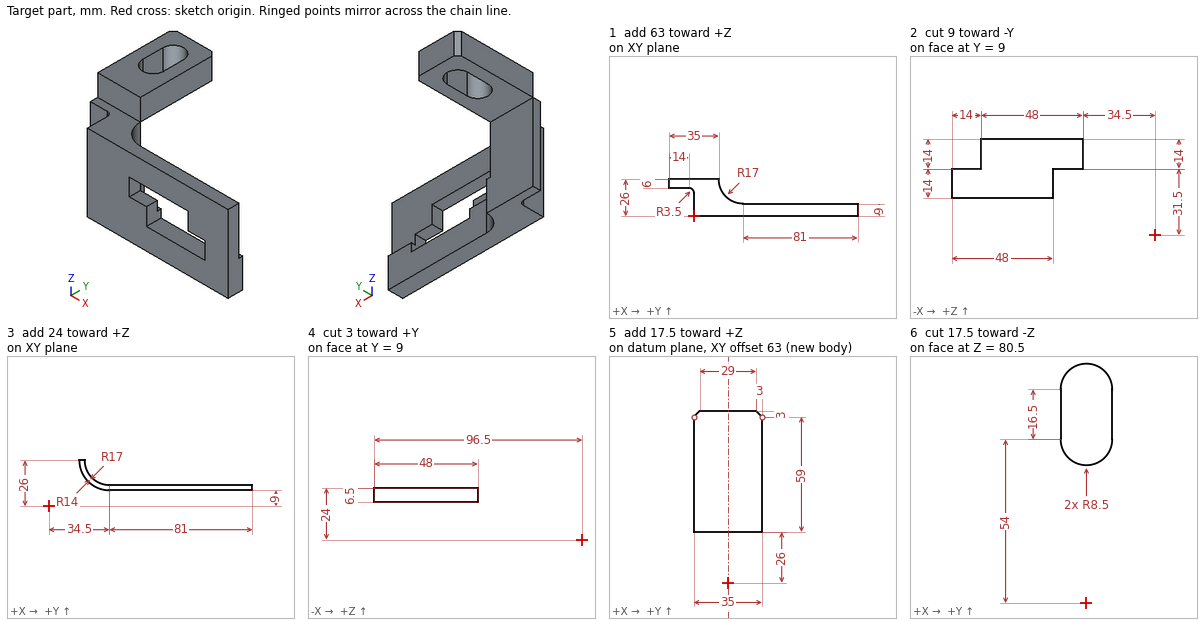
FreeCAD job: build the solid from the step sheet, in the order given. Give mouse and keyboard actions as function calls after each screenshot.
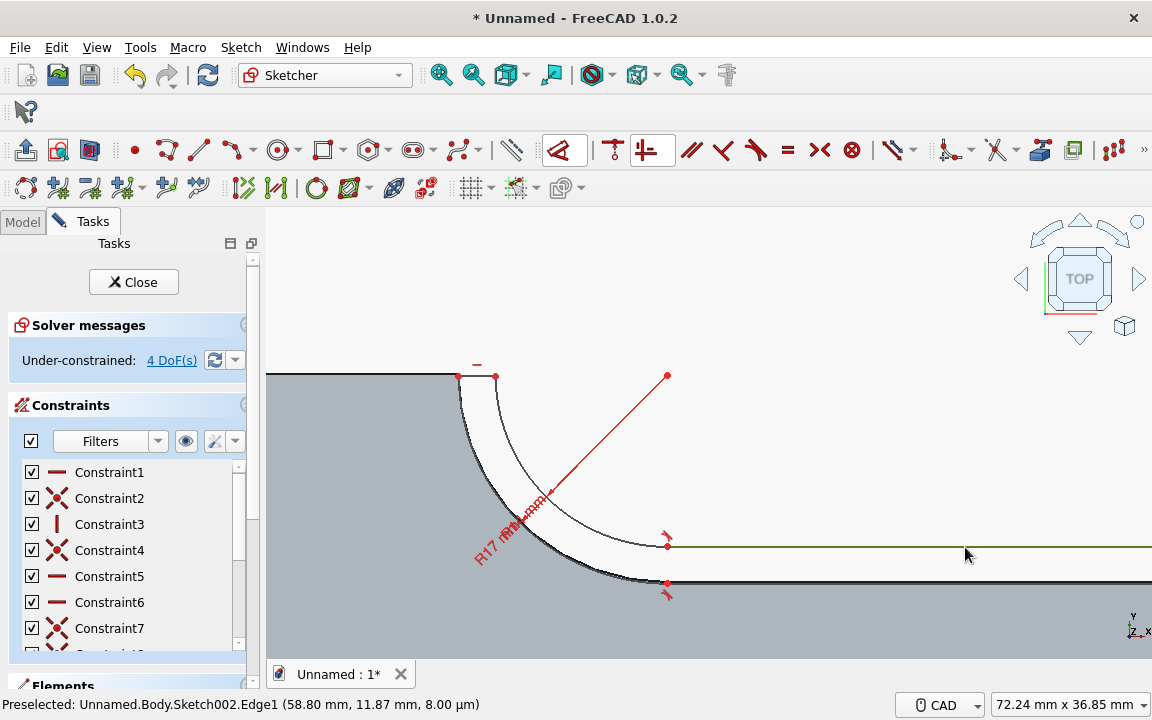
key(l)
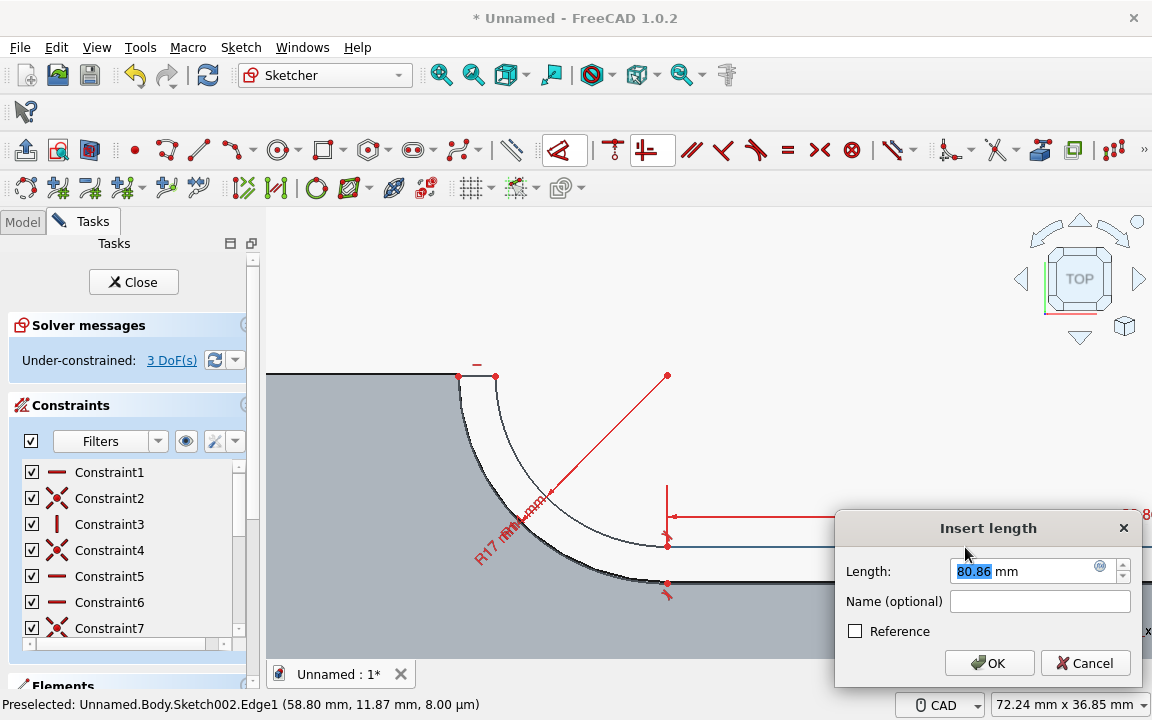
text(81)
key(Return)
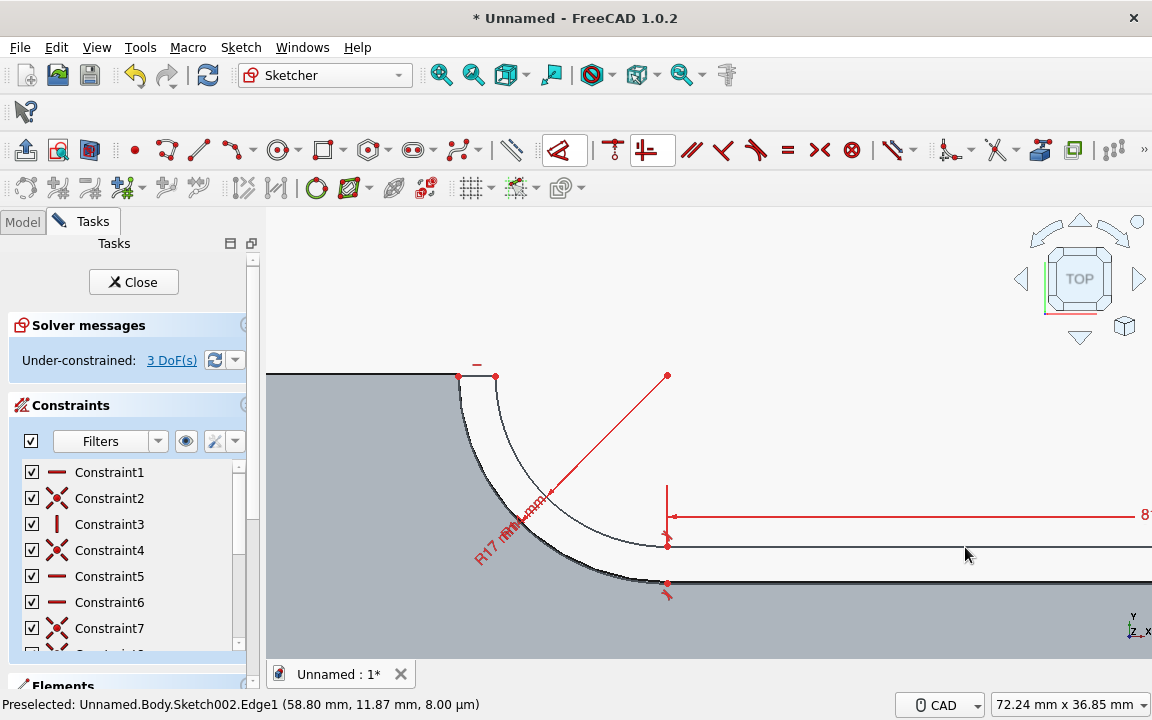
scroll(459, 375, down, 5)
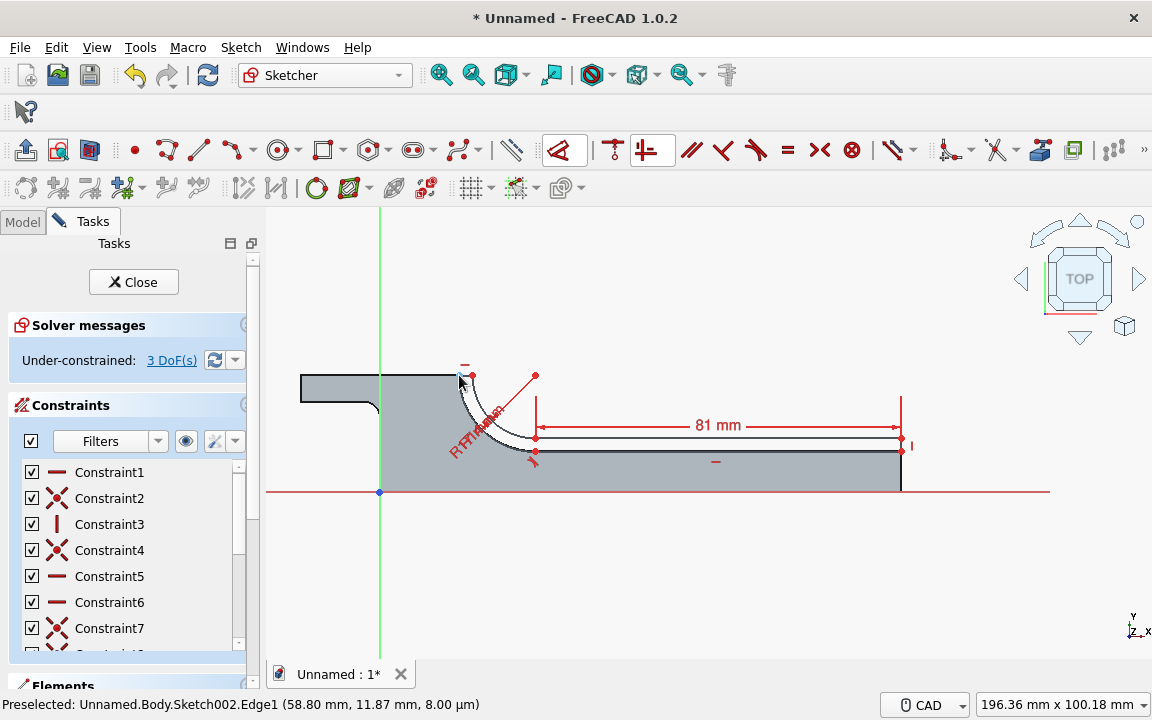
click(901, 452)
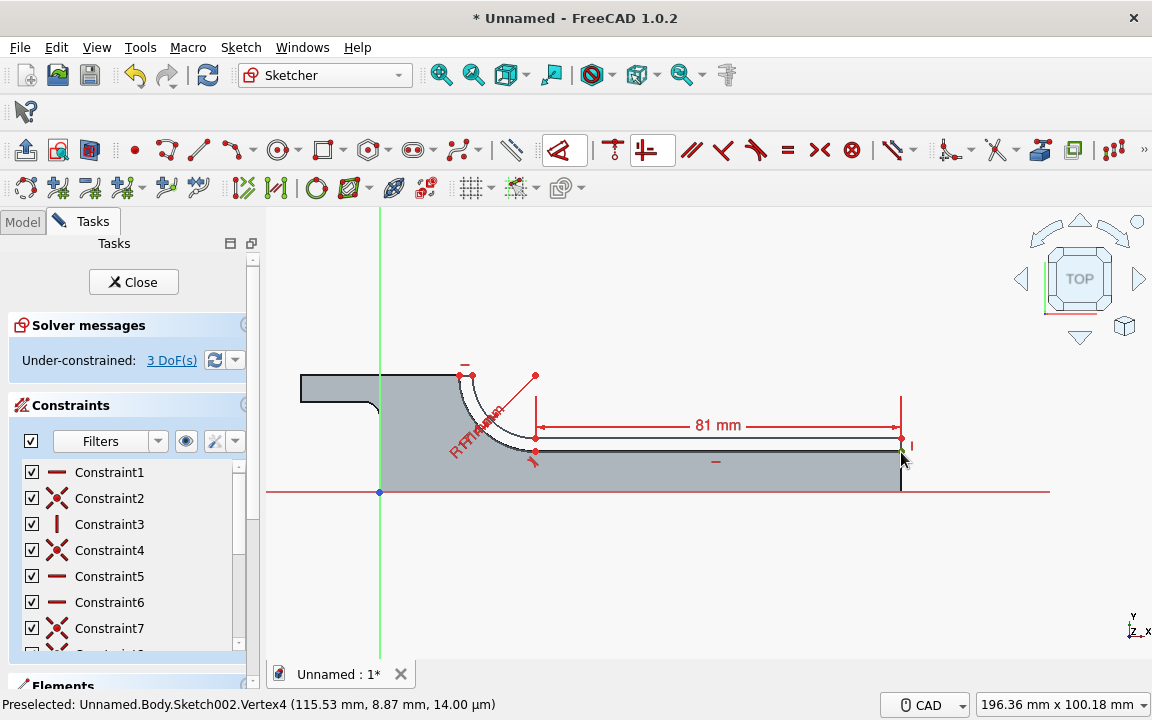
key(i)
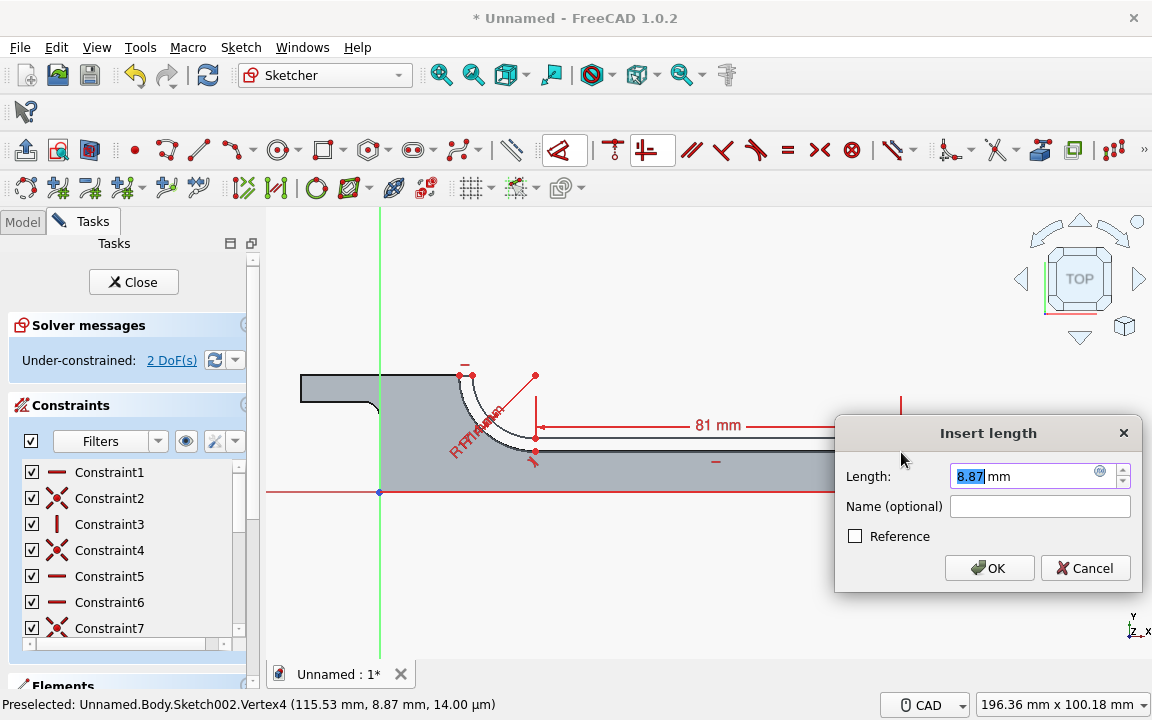
text(9)
key(Return)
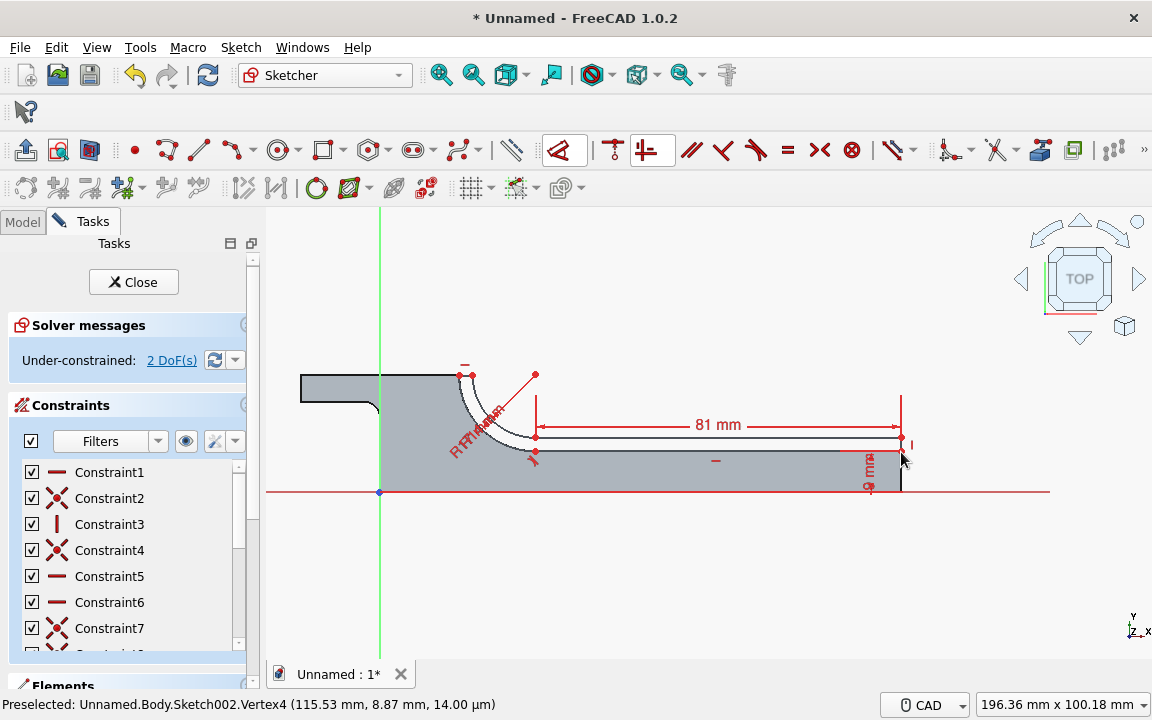
click(459, 376)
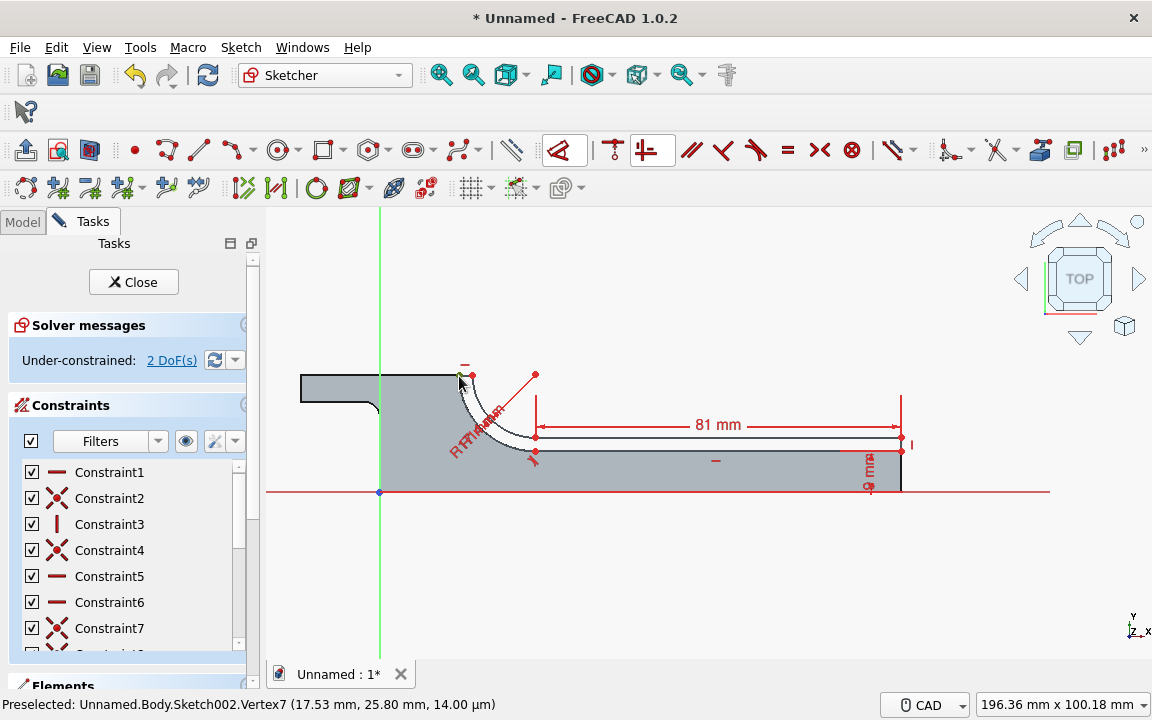
key(i)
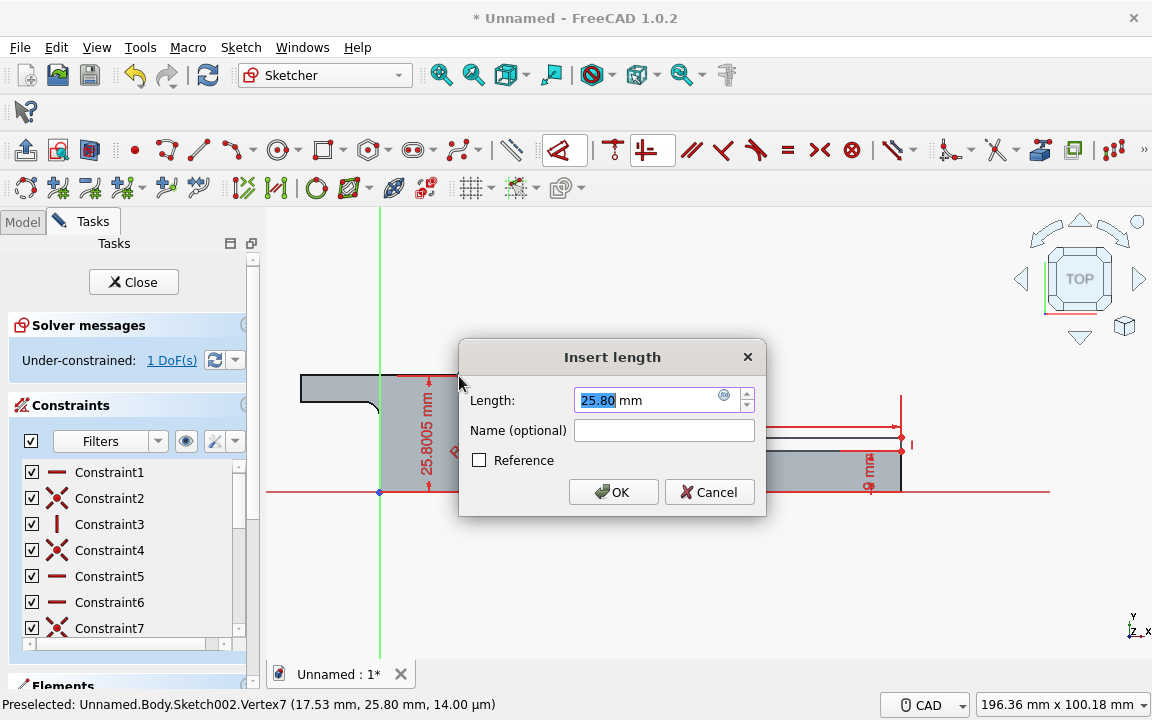
text(26)
key(Return)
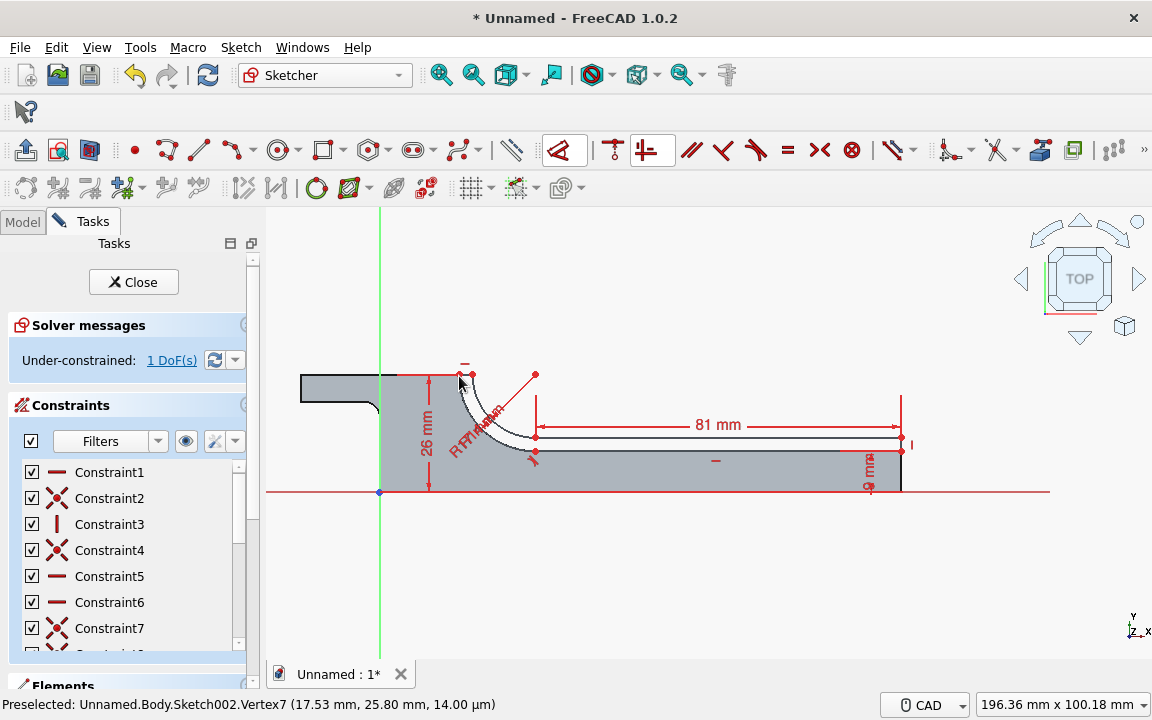
click(536, 438)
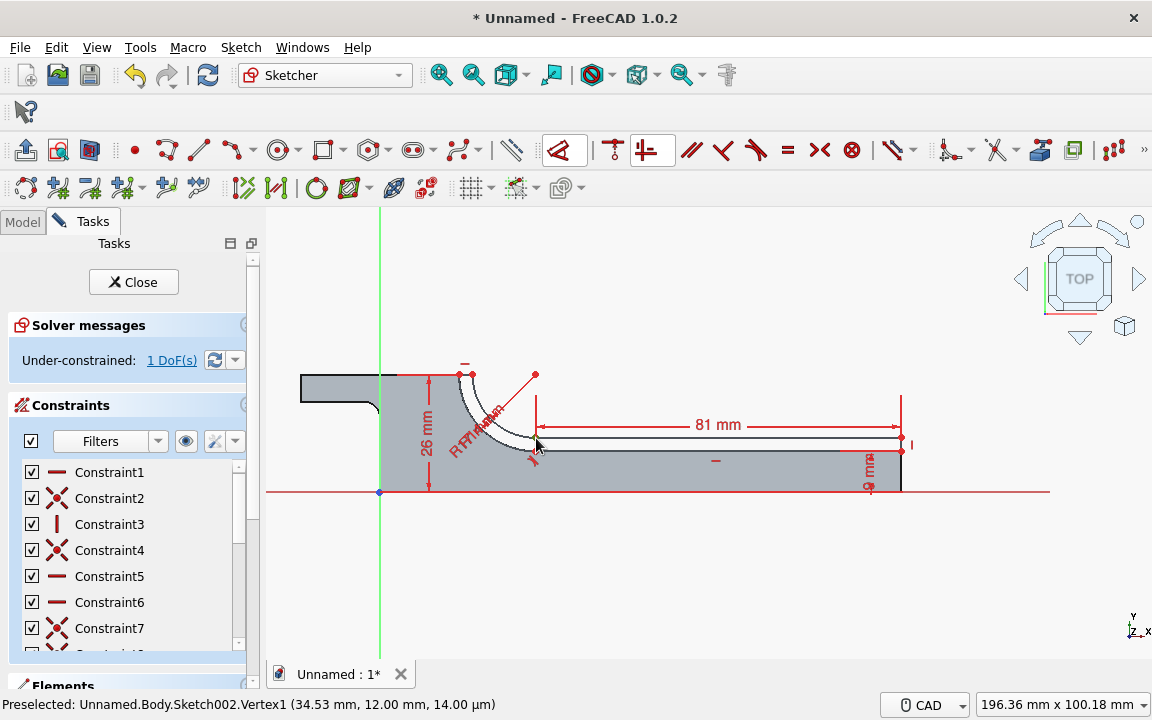
key(l)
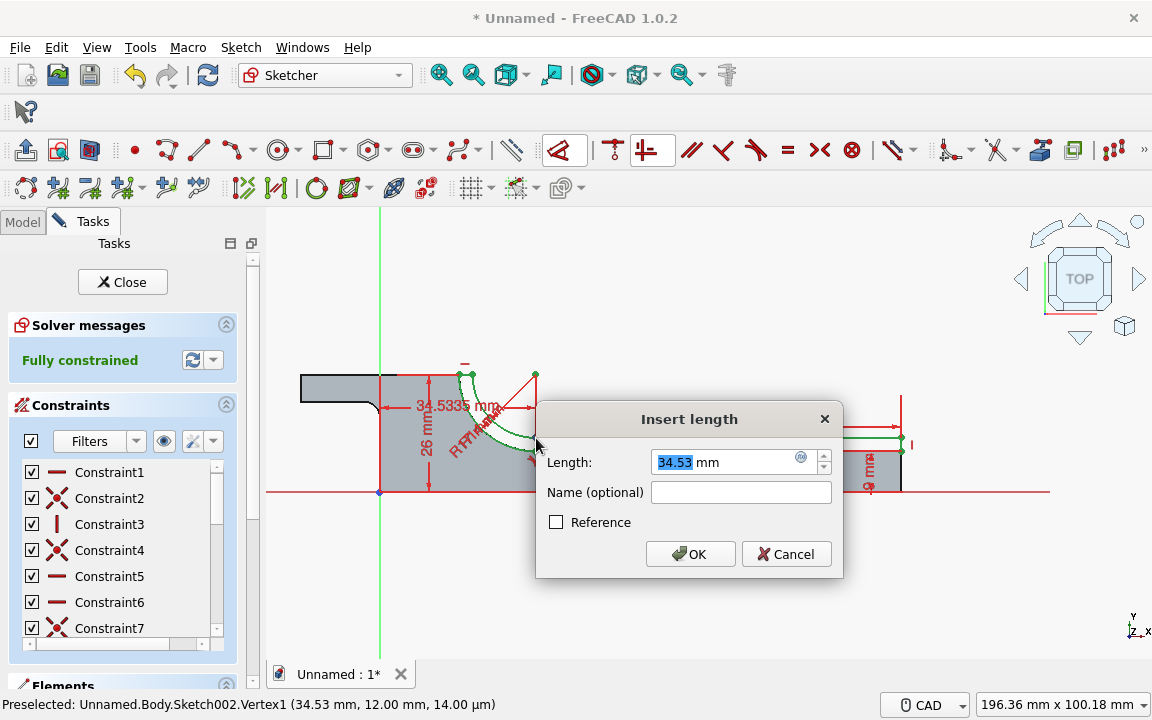
text(34.5)
key(Return)